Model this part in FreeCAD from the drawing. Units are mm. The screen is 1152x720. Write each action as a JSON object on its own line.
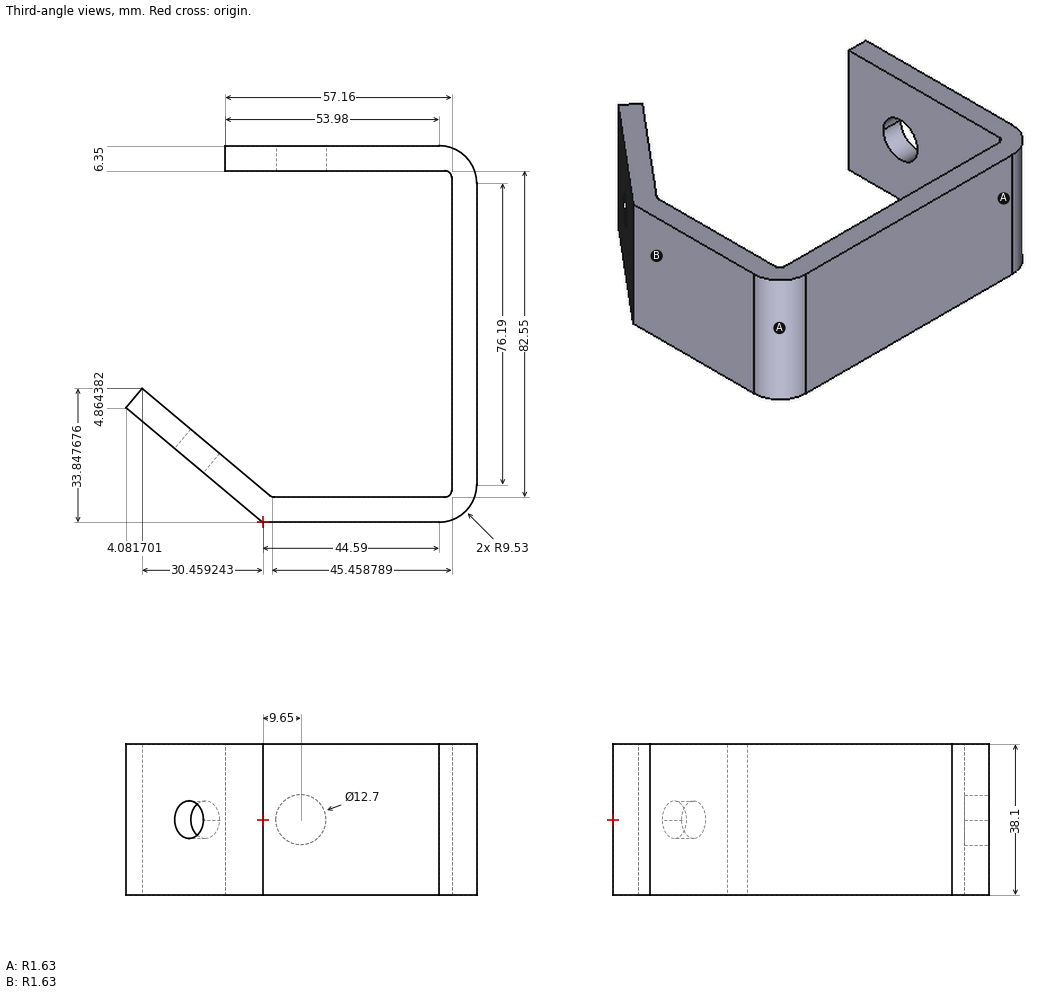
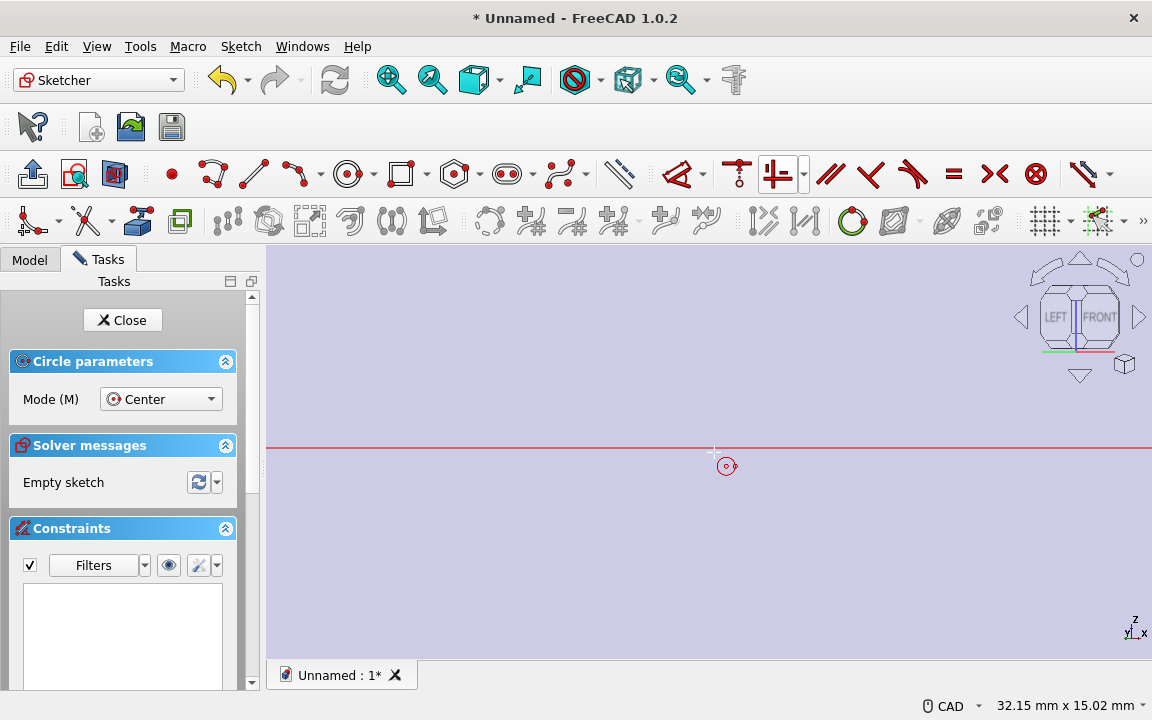
{"action": "left_click", "coordinate": [633, 448]}
{"action": "mouse_move", "coordinate": [726, 355]}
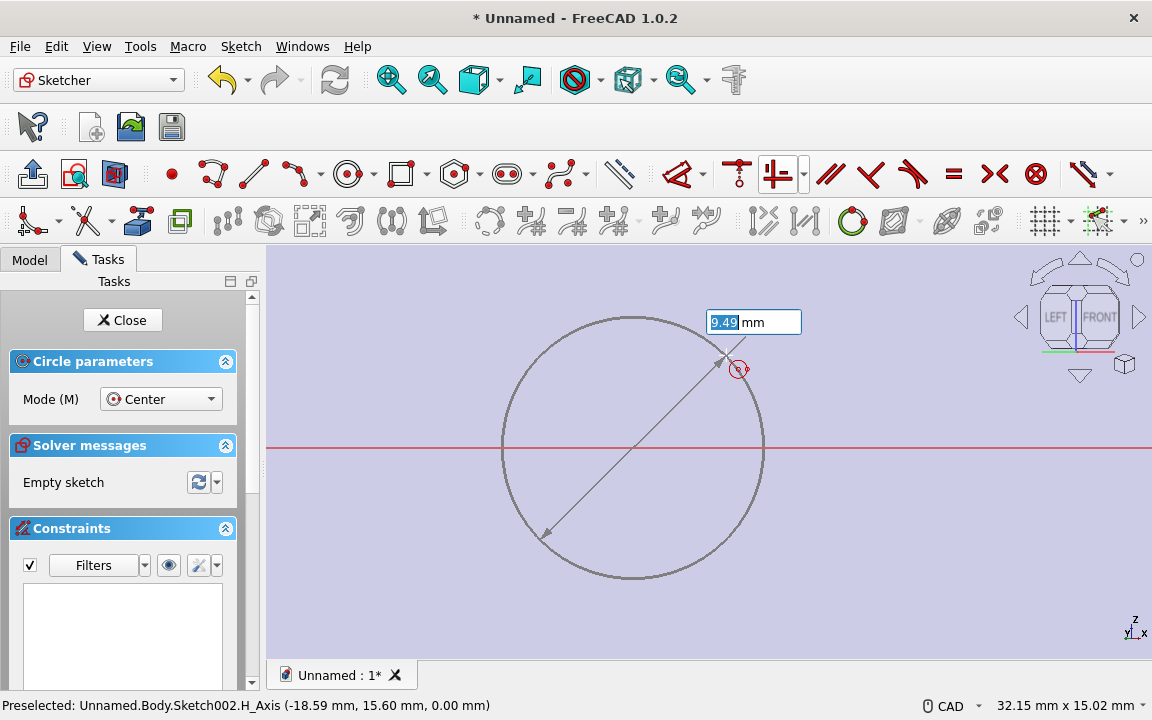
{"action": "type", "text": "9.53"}
{"action": "key", "text": "Return"}
{"action": "key", "text": "Escape"}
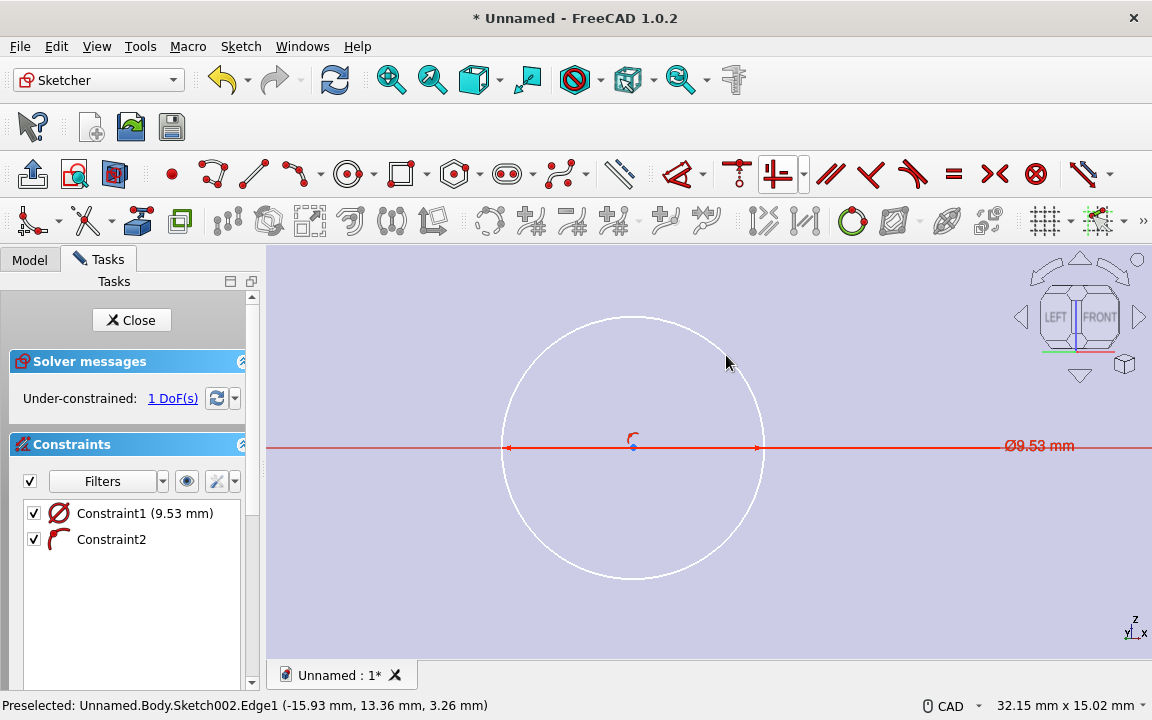
{"action": "key", "text": "d"}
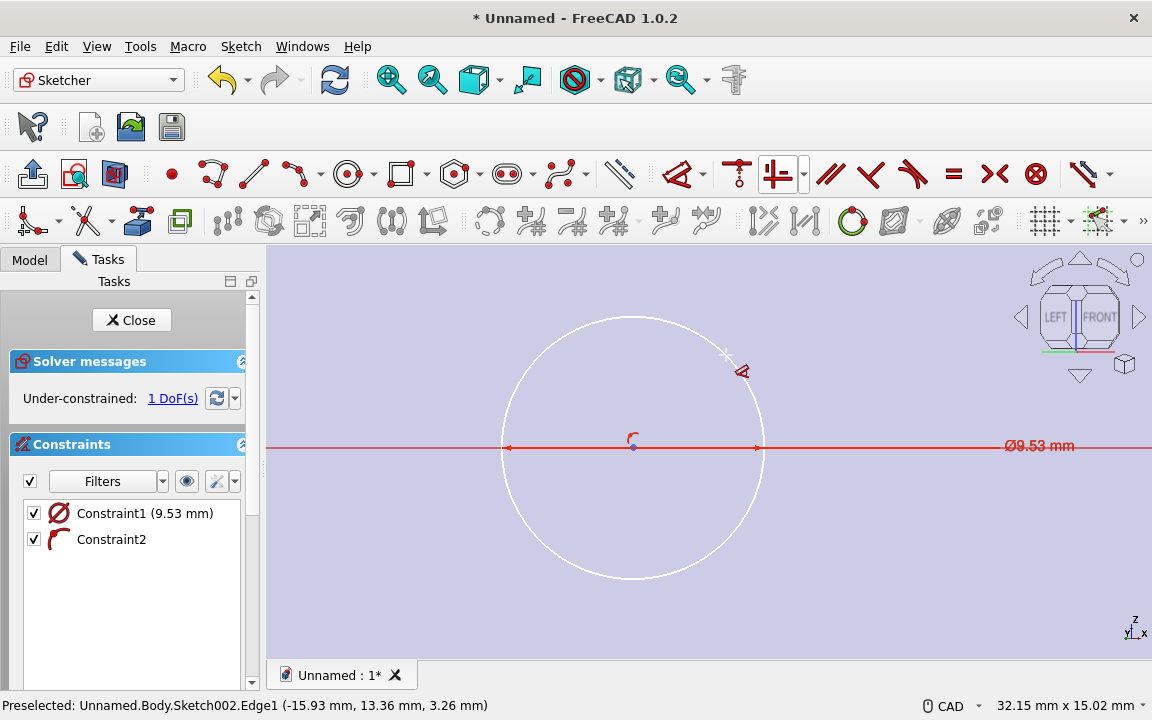
{"action": "left_click", "coordinate": [633, 448]}
{"action": "left_click", "coordinate": [810, 482]}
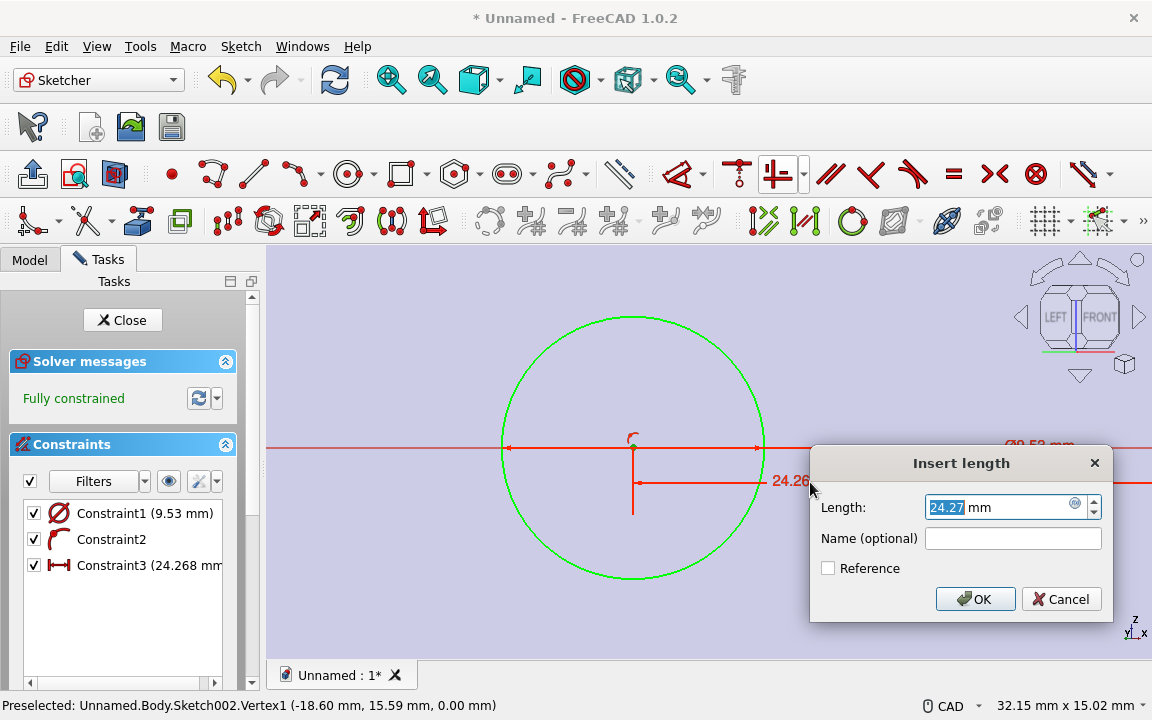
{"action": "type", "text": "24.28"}
{"action": "key", "text": "Return"}
{"action": "key", "text": "Escape"}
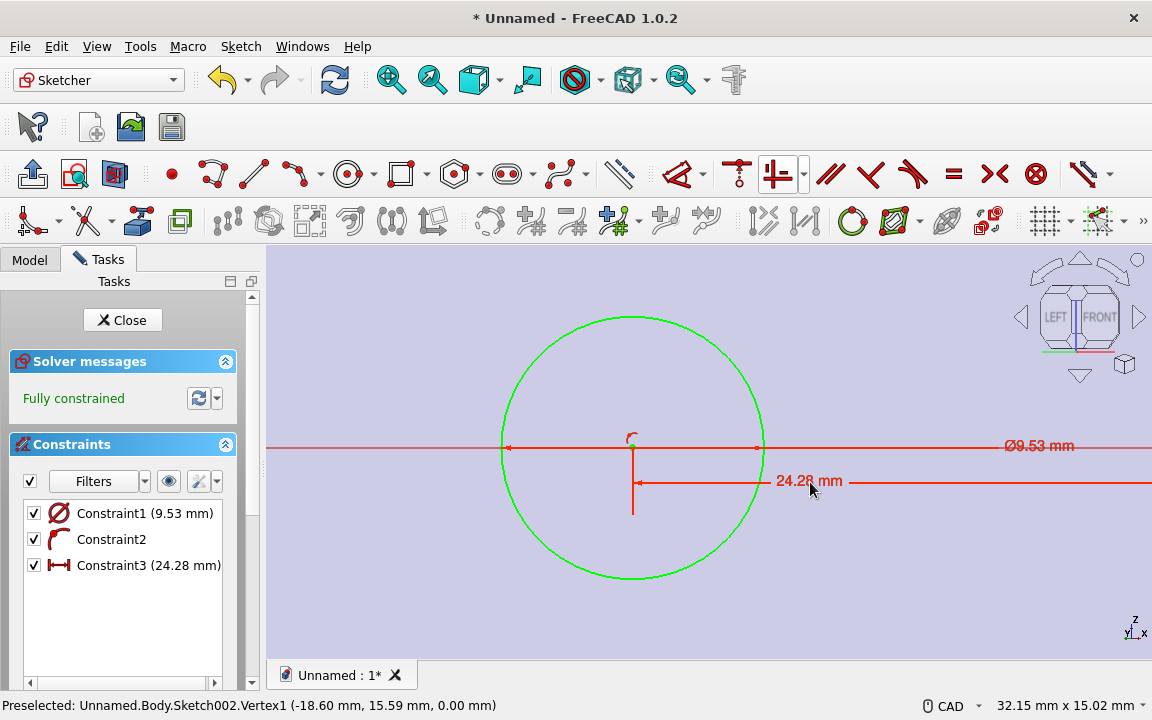
{"action": "left_click", "coordinate": [123, 320]}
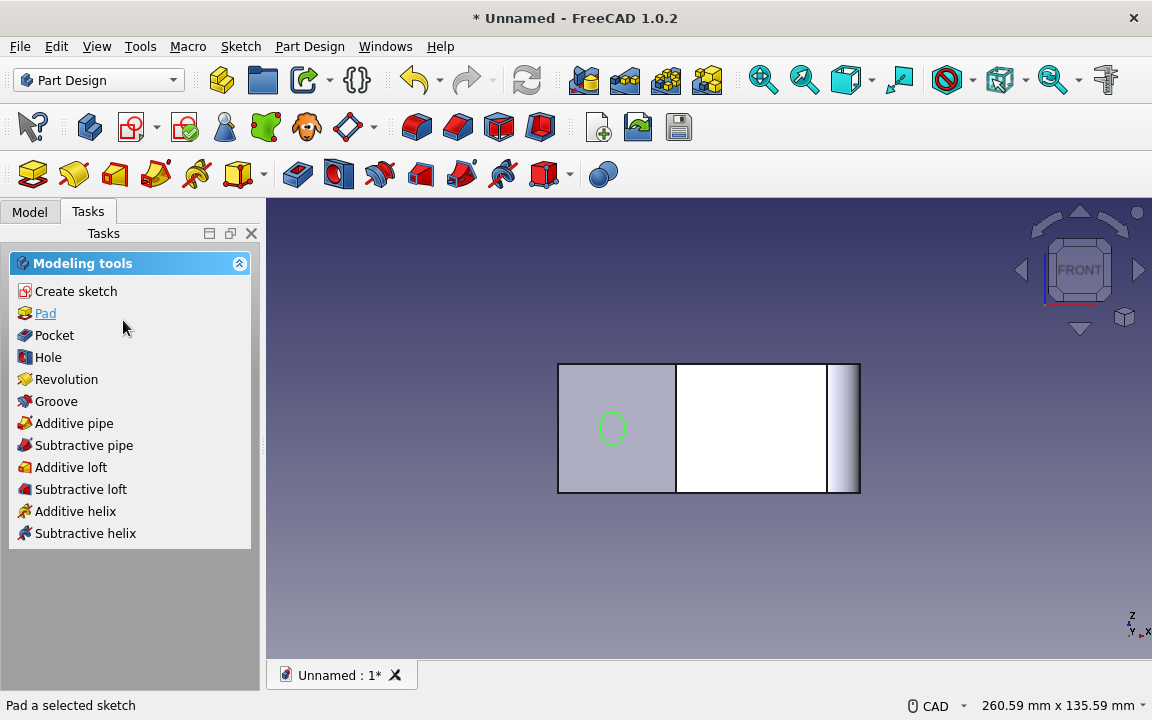
{"action": "left_click", "coordinate": [298, 174]}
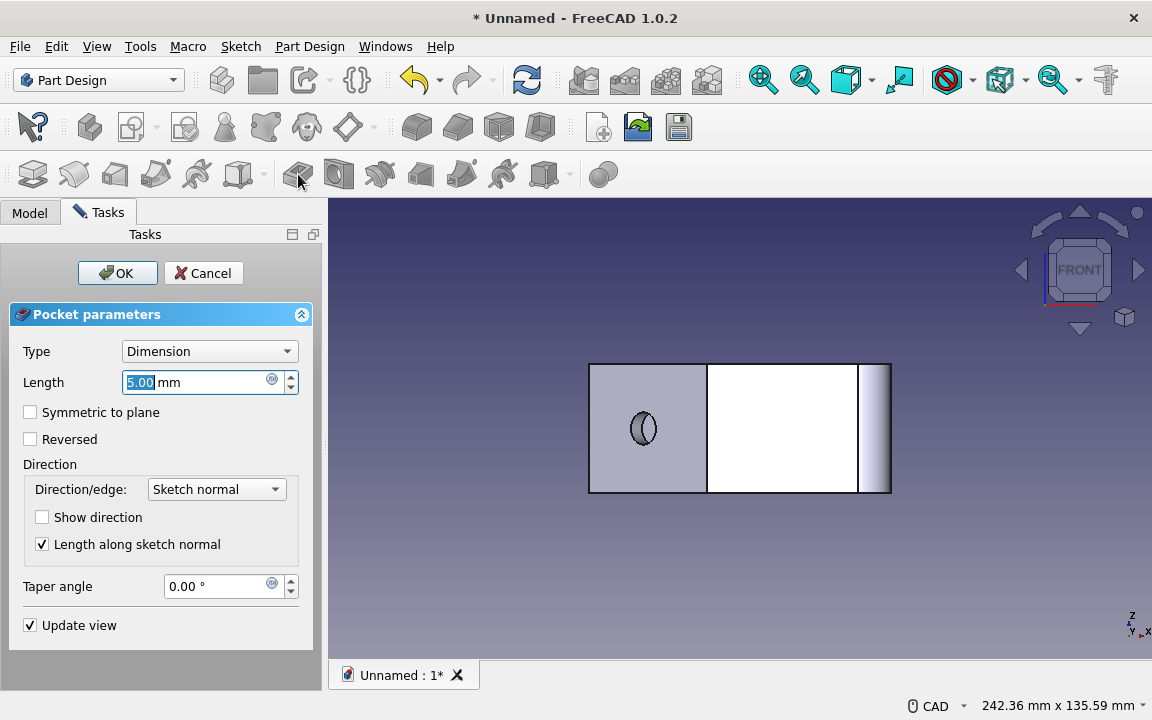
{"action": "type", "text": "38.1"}
{"action": "key", "text": "Tab"}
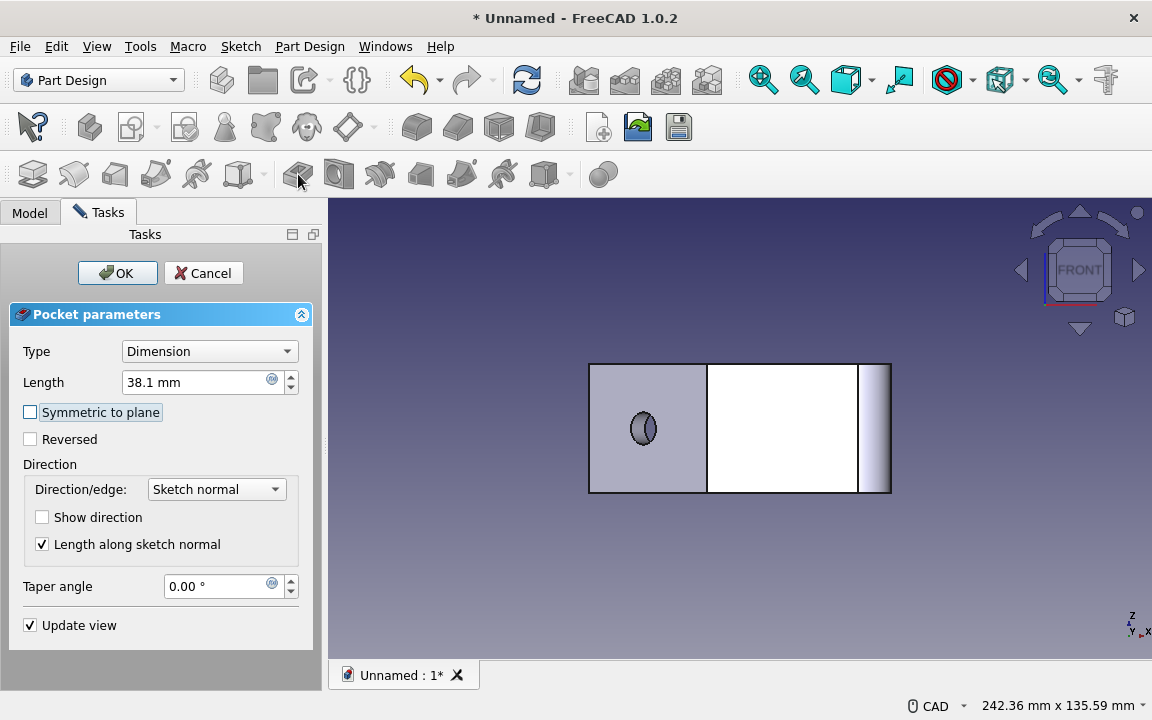
{"action": "left_click", "coordinate": [31, 412]}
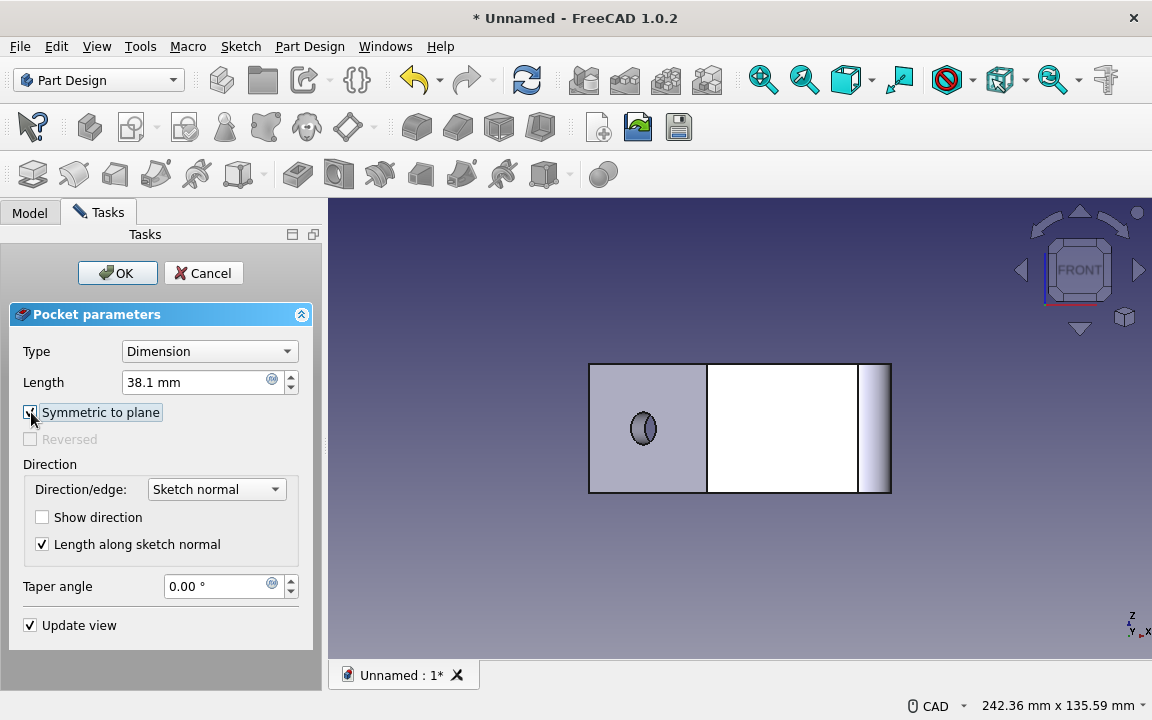
{"action": "left_click", "coordinate": [118, 273]}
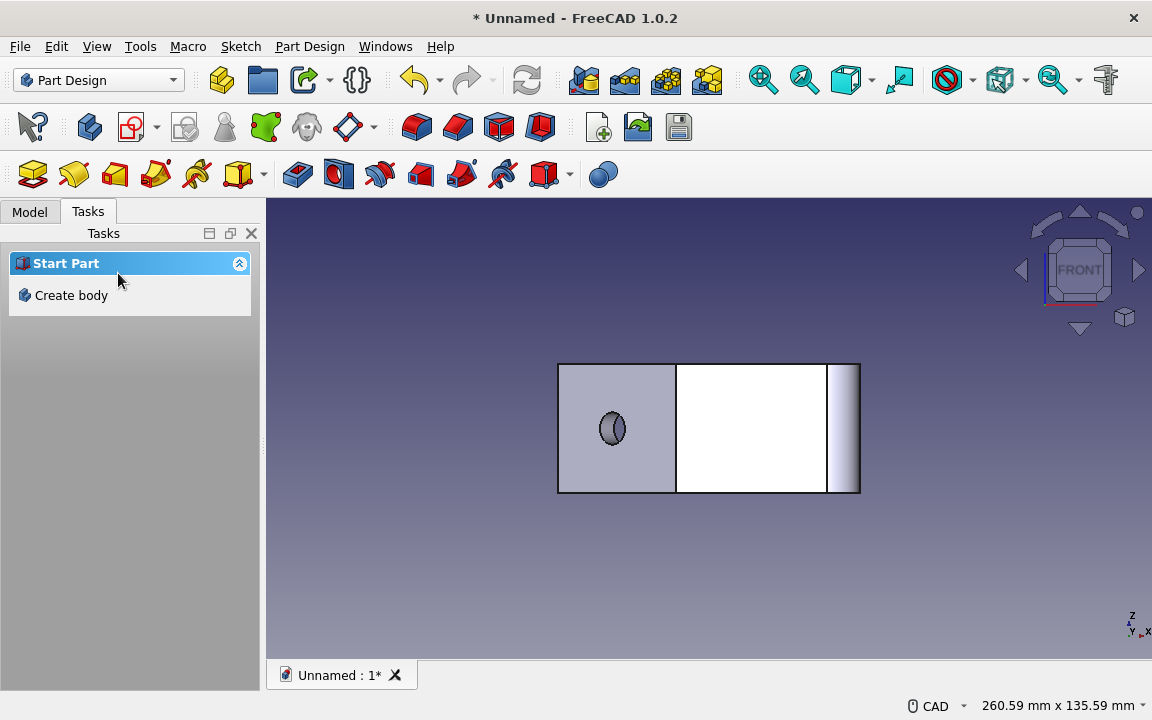
{"action": "key", "text": "v f"}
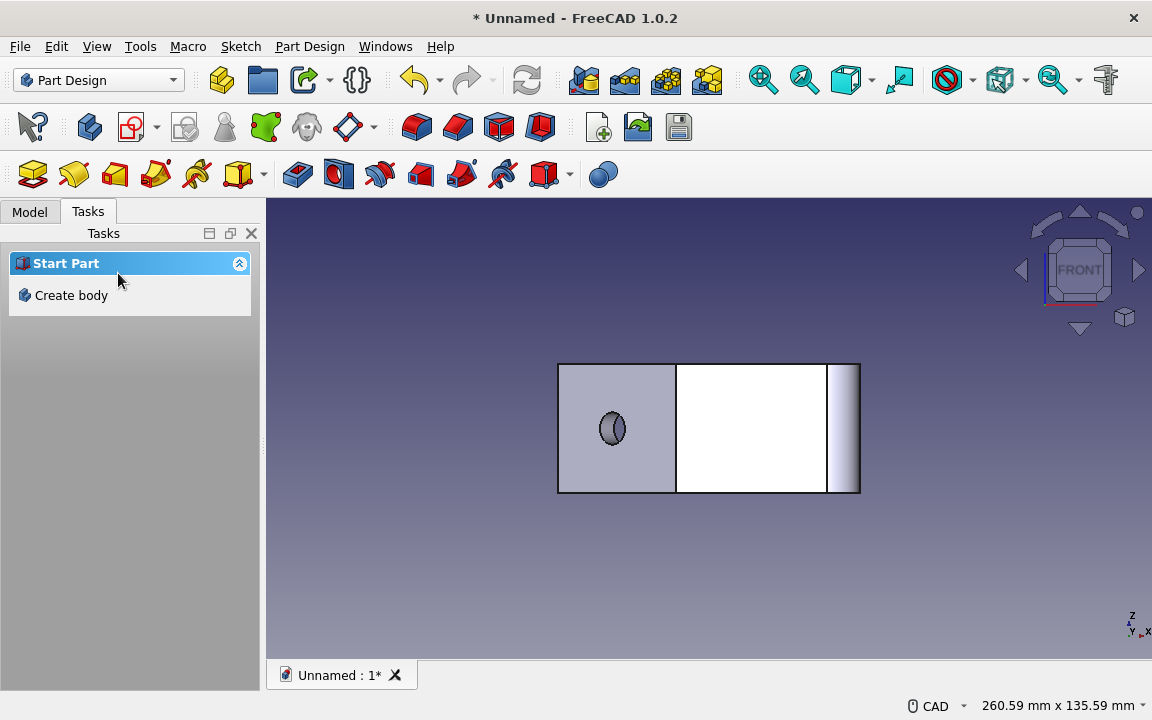
{"action": "key", "text": "0"}